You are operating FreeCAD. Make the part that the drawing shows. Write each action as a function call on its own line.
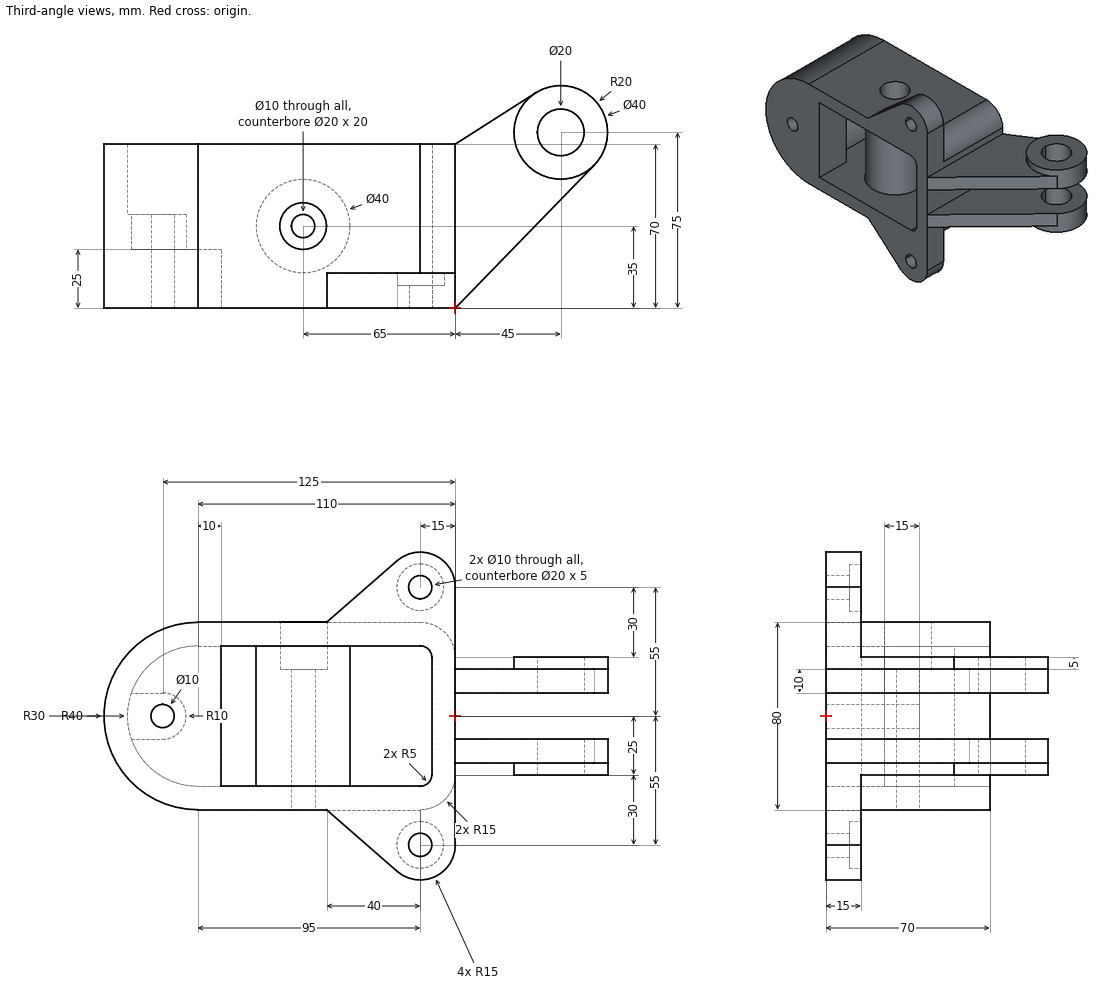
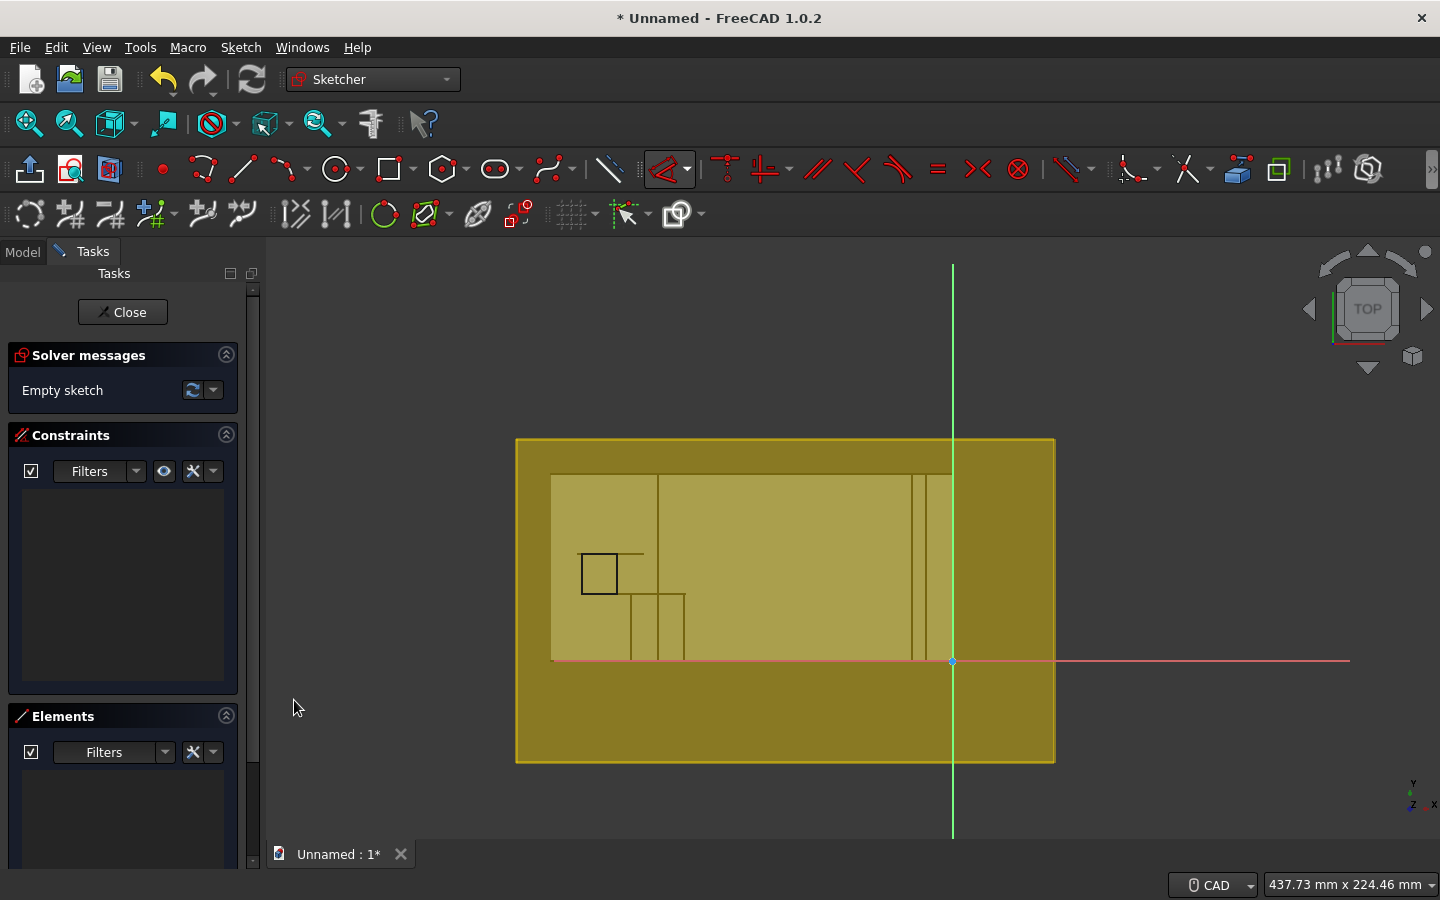
scroll(1275, 539, up, 2)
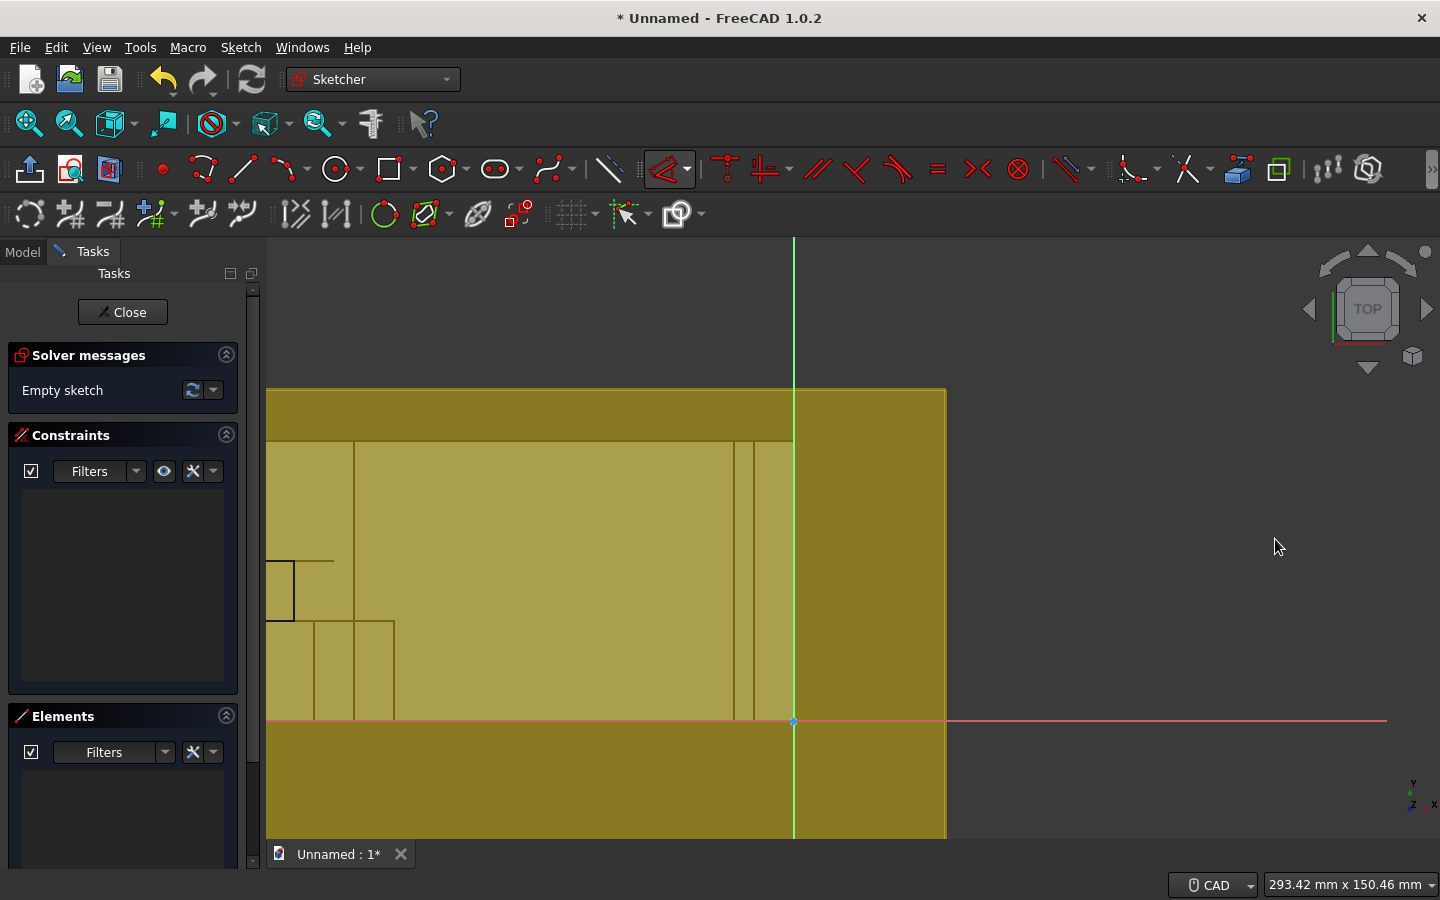
key(g)
key(m)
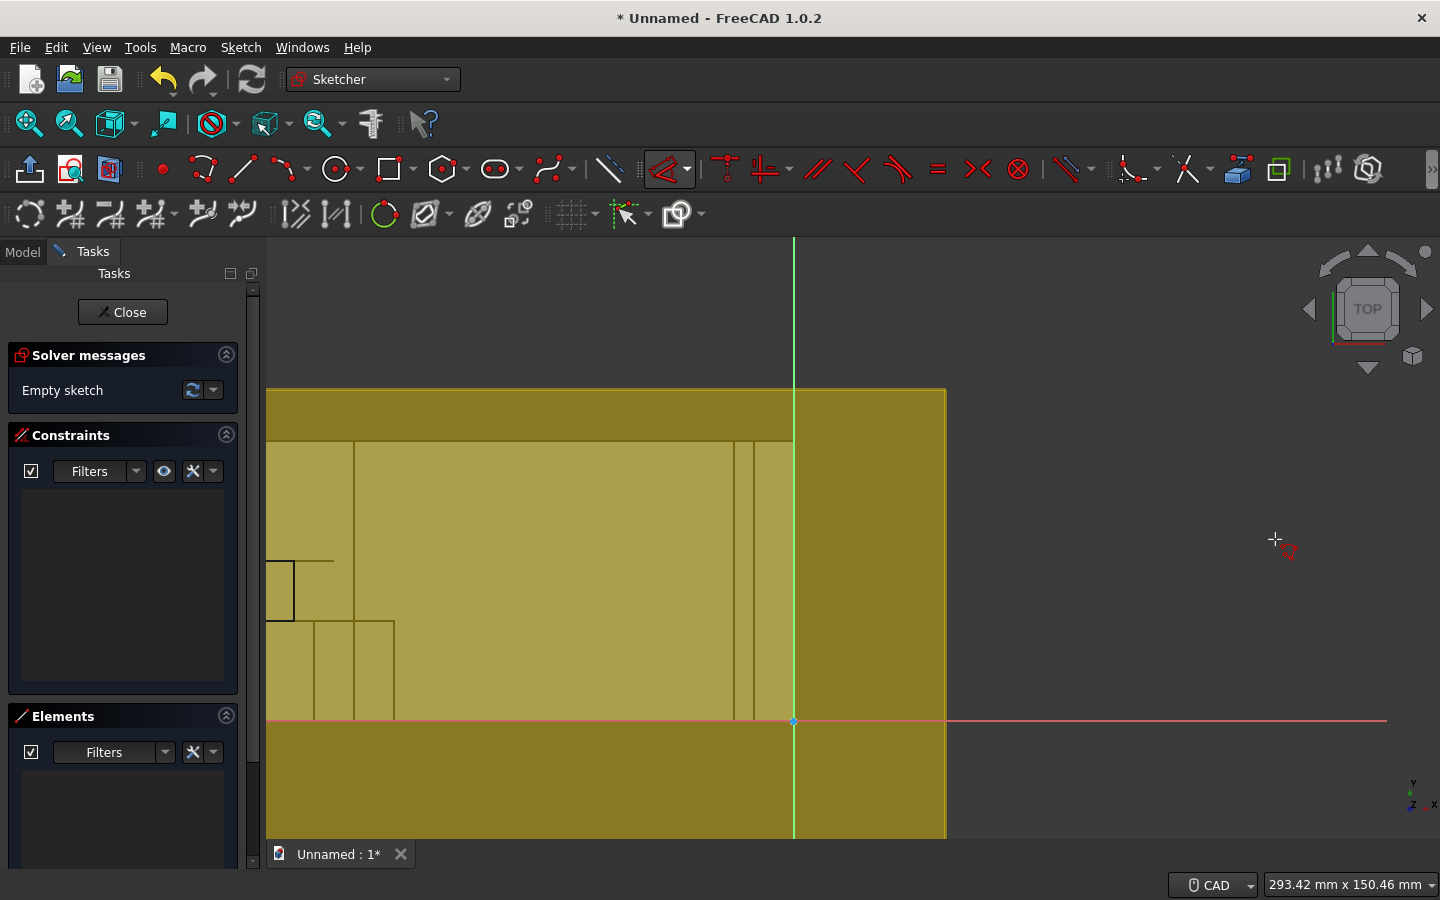
click(931, 354)
click(794, 441)
click(794, 721)
click(1031, 477)
right_click(1031, 477)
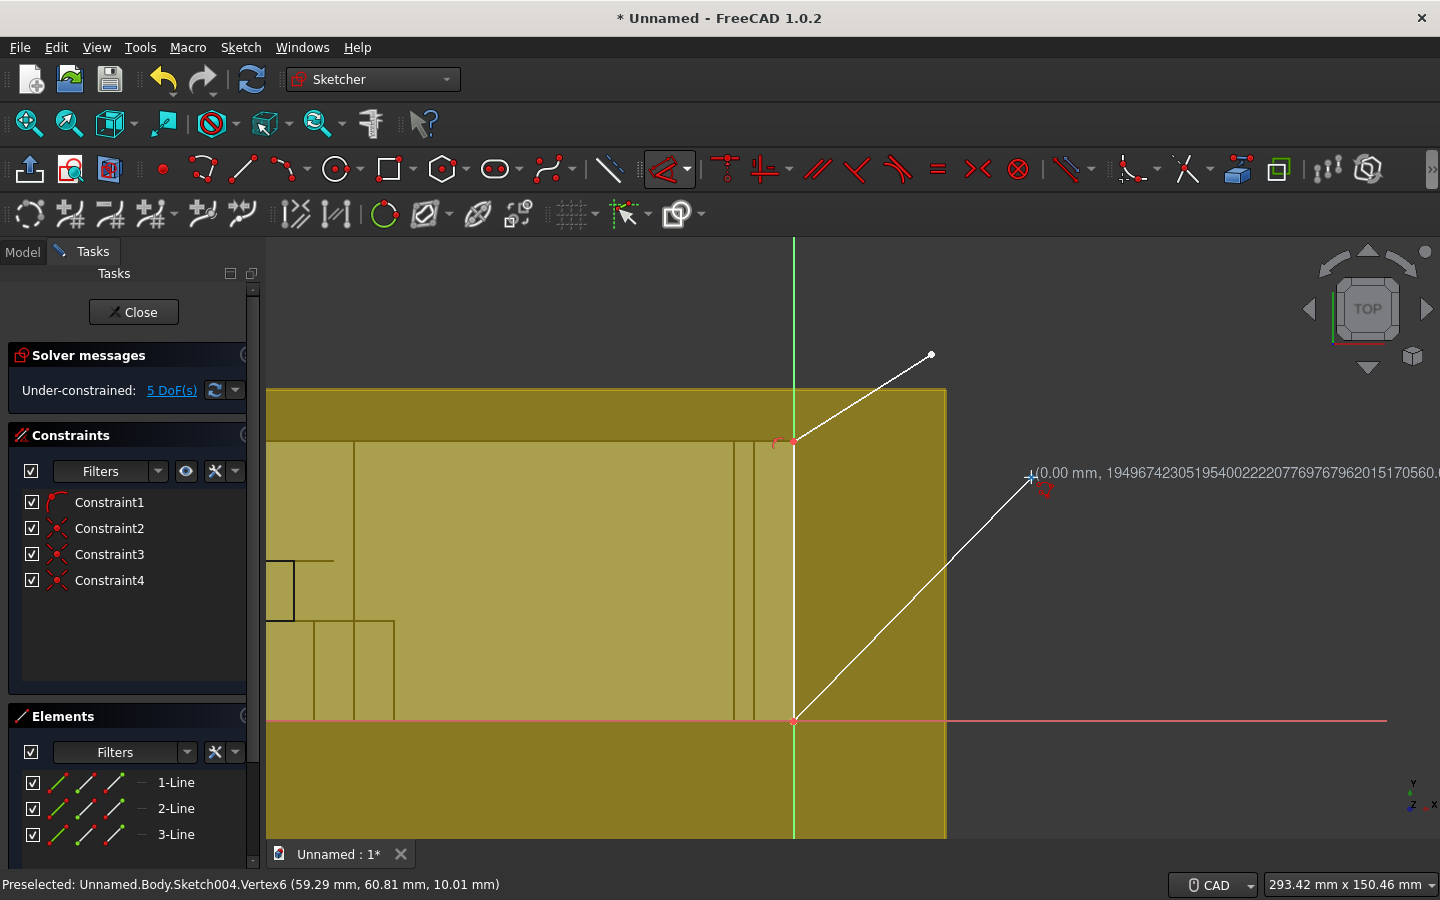
key(g)
key(3)
key(a)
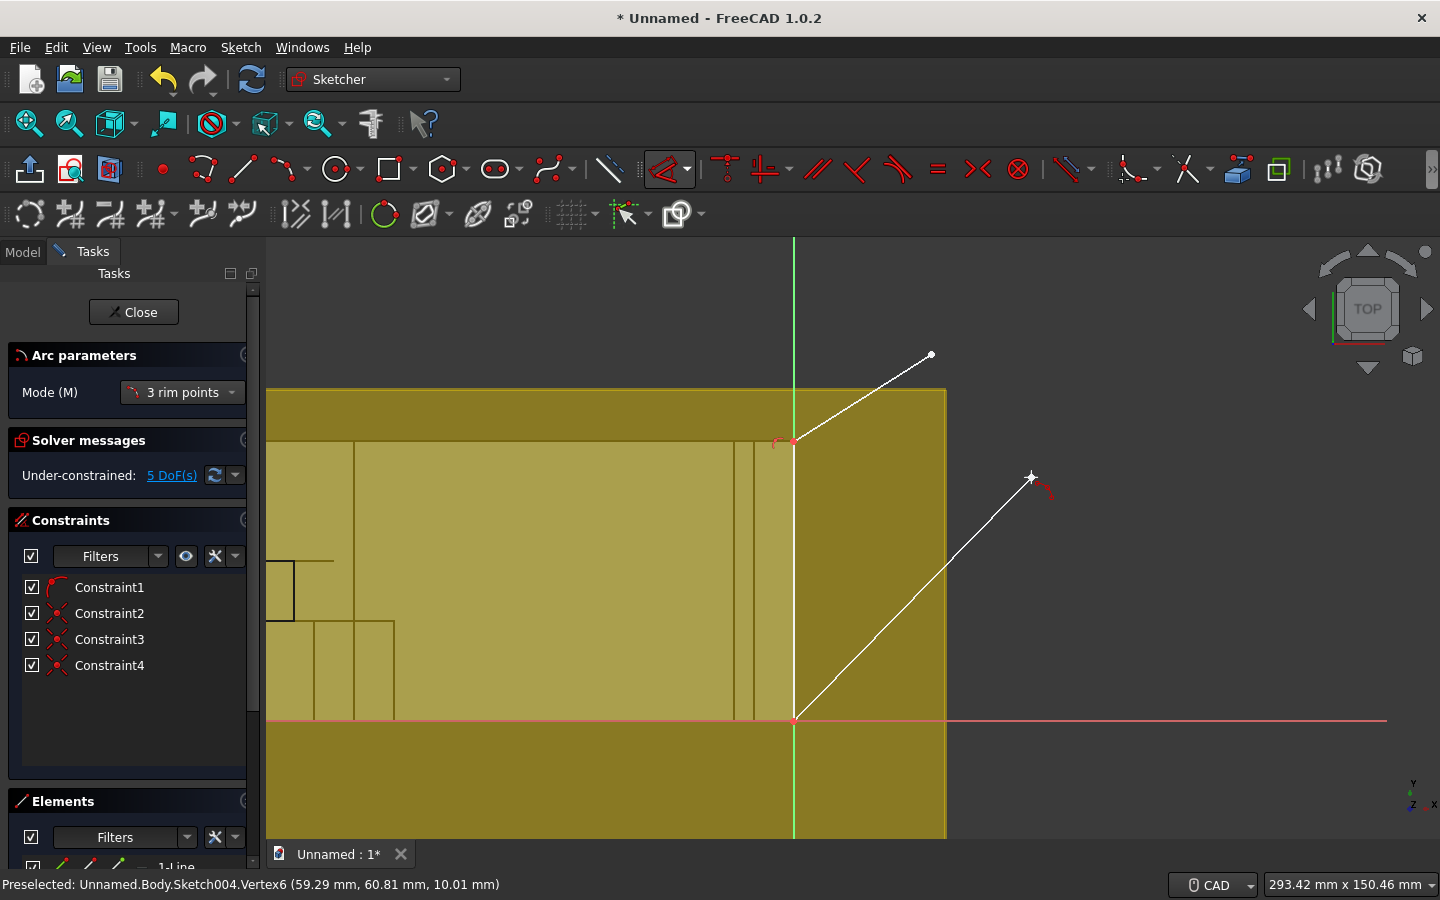
click(1031, 478)
click(931, 355)
click(1036, 371)
key(Escape)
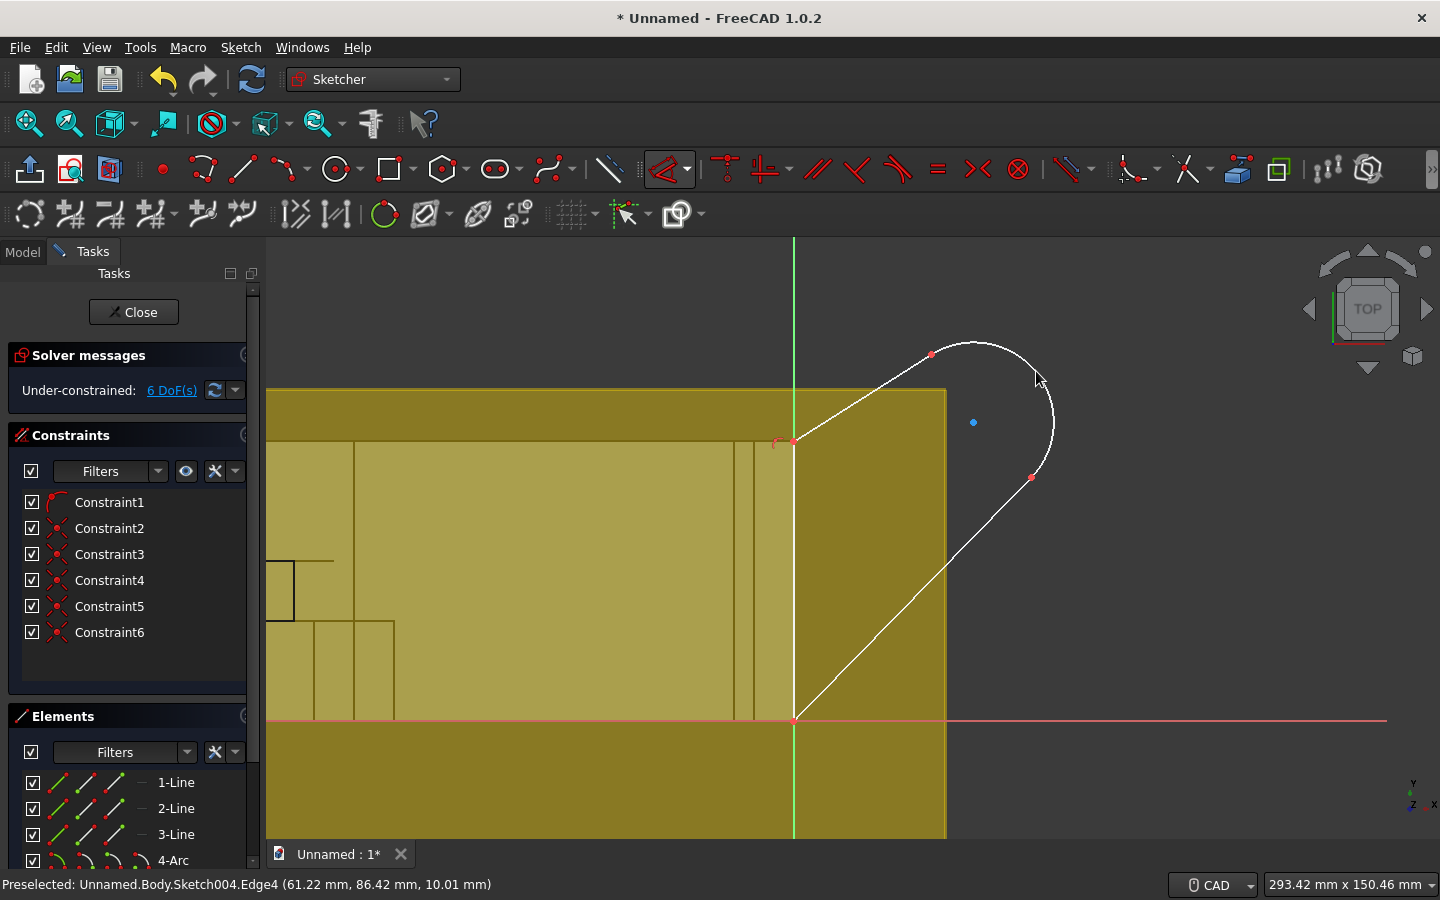
click(890, 381)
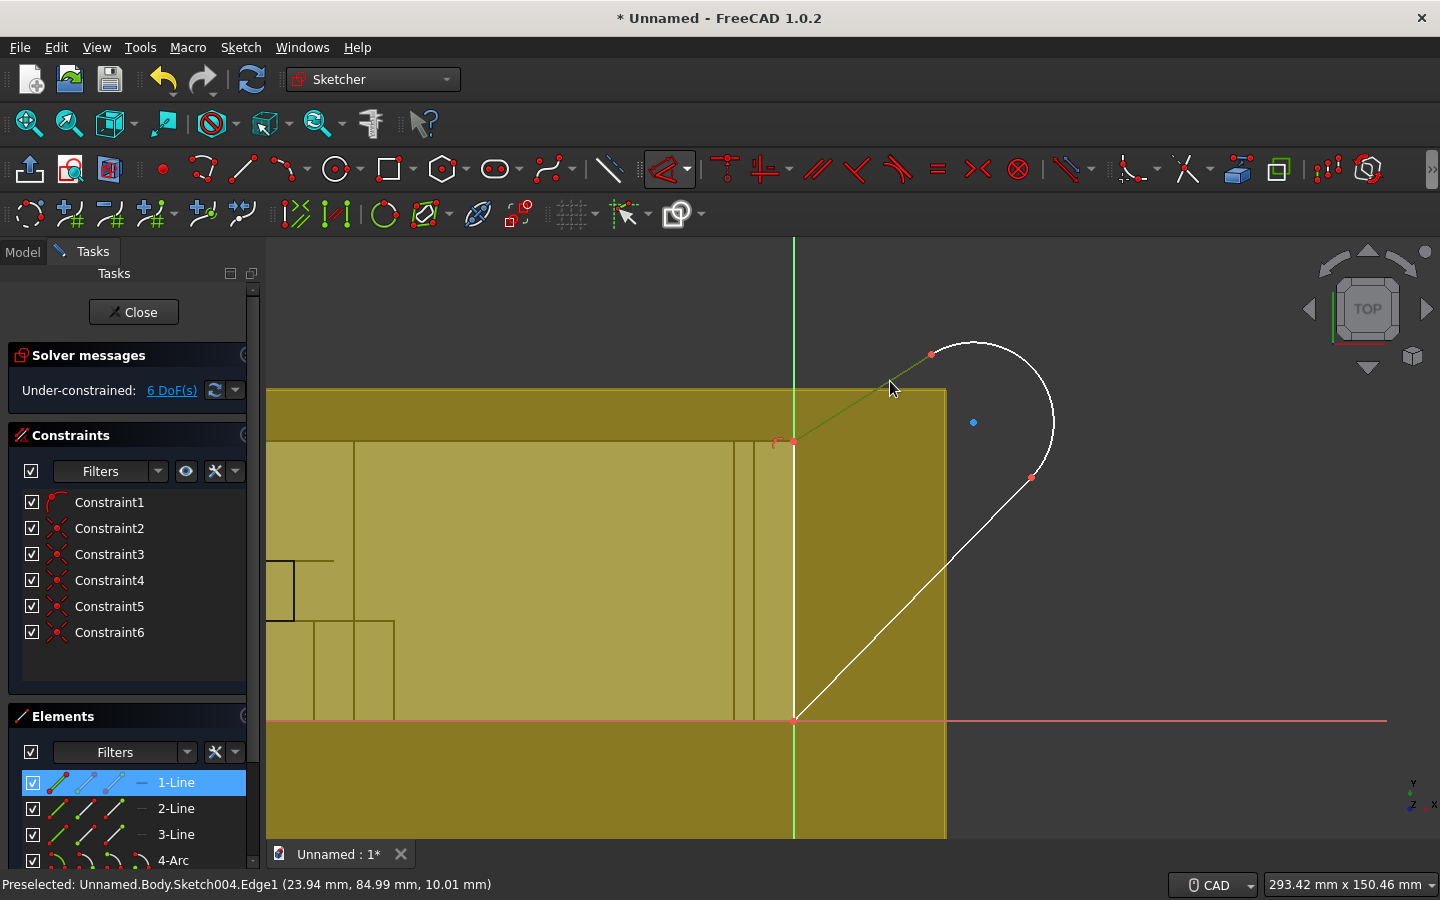
click(1053, 414)